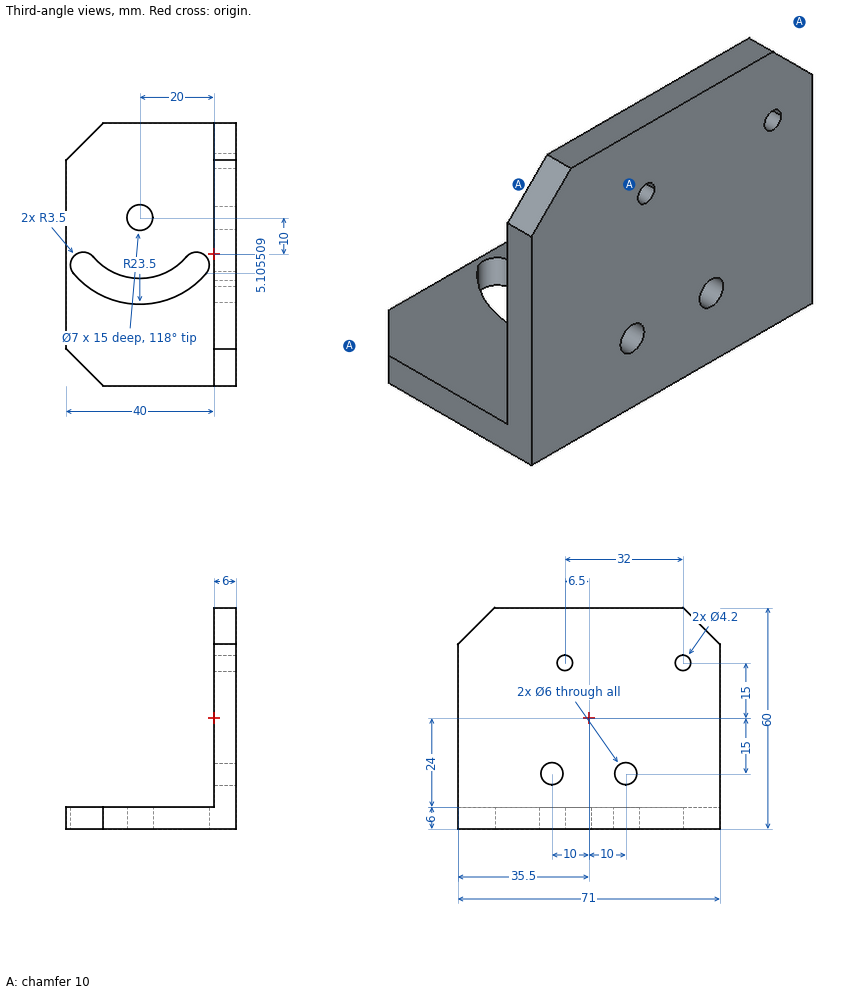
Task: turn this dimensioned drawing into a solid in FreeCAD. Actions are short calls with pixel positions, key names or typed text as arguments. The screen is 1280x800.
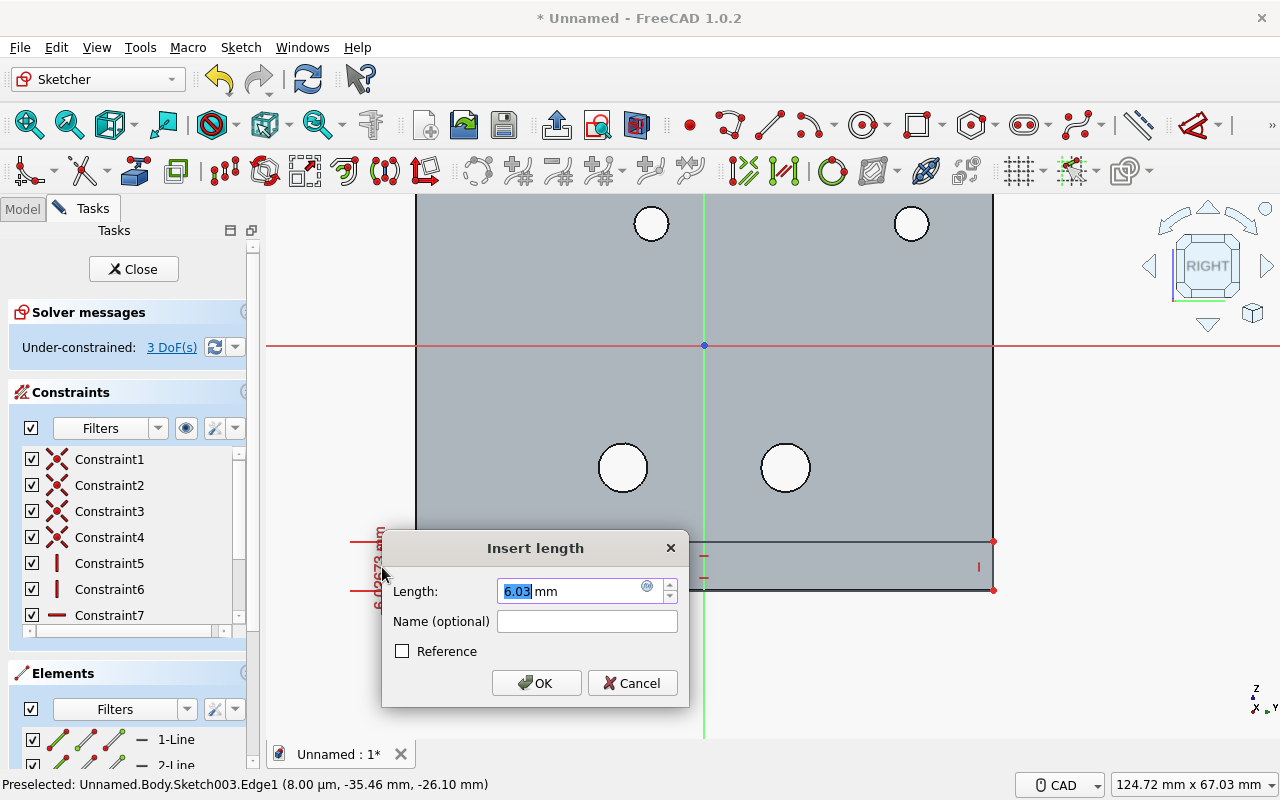
text(6)
key(Return)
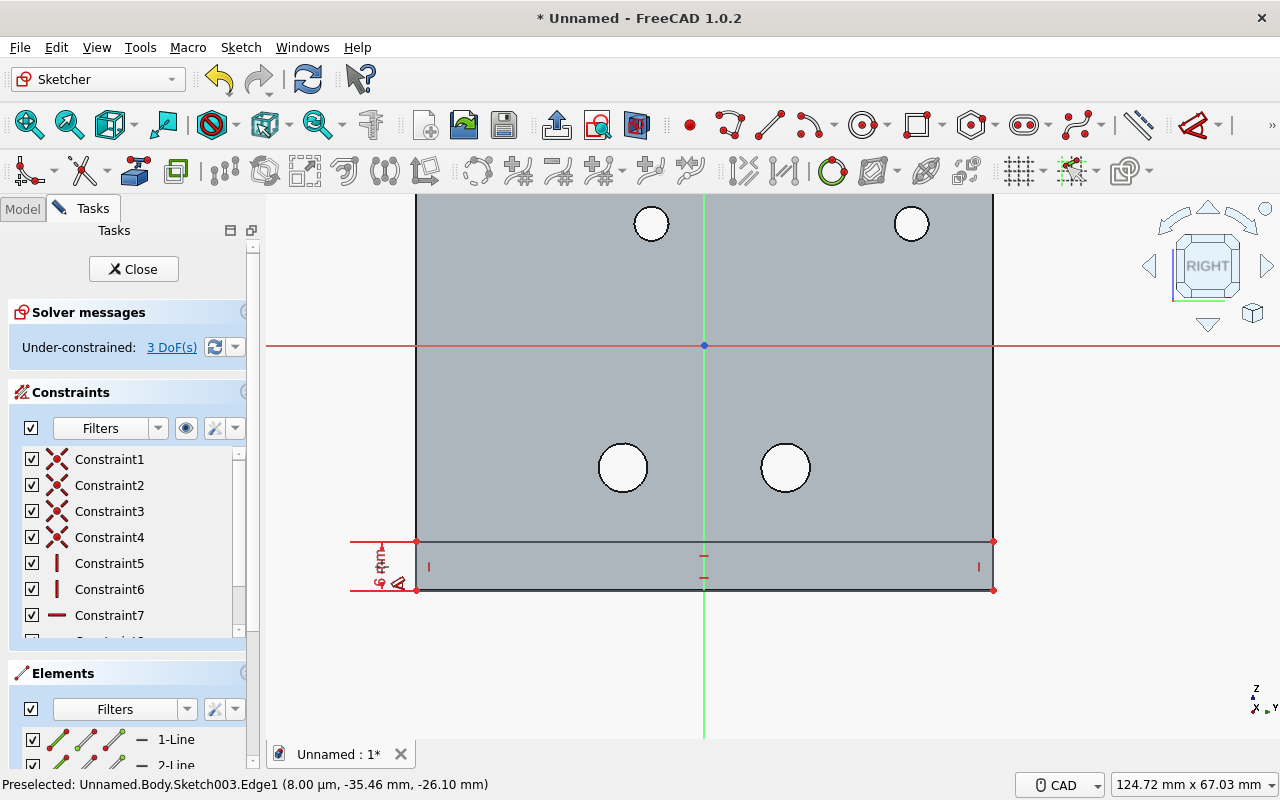
click(589, 591)
click(572, 625)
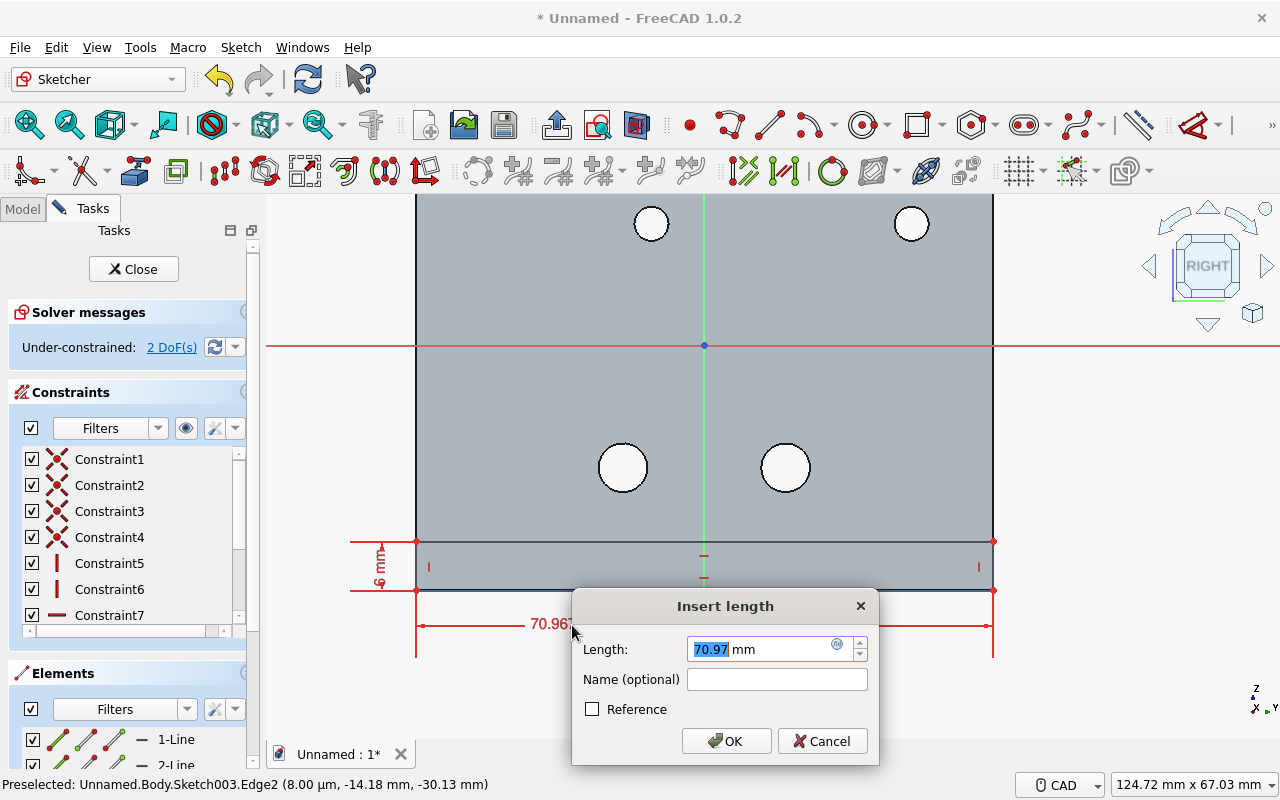
text(71)
key(Return)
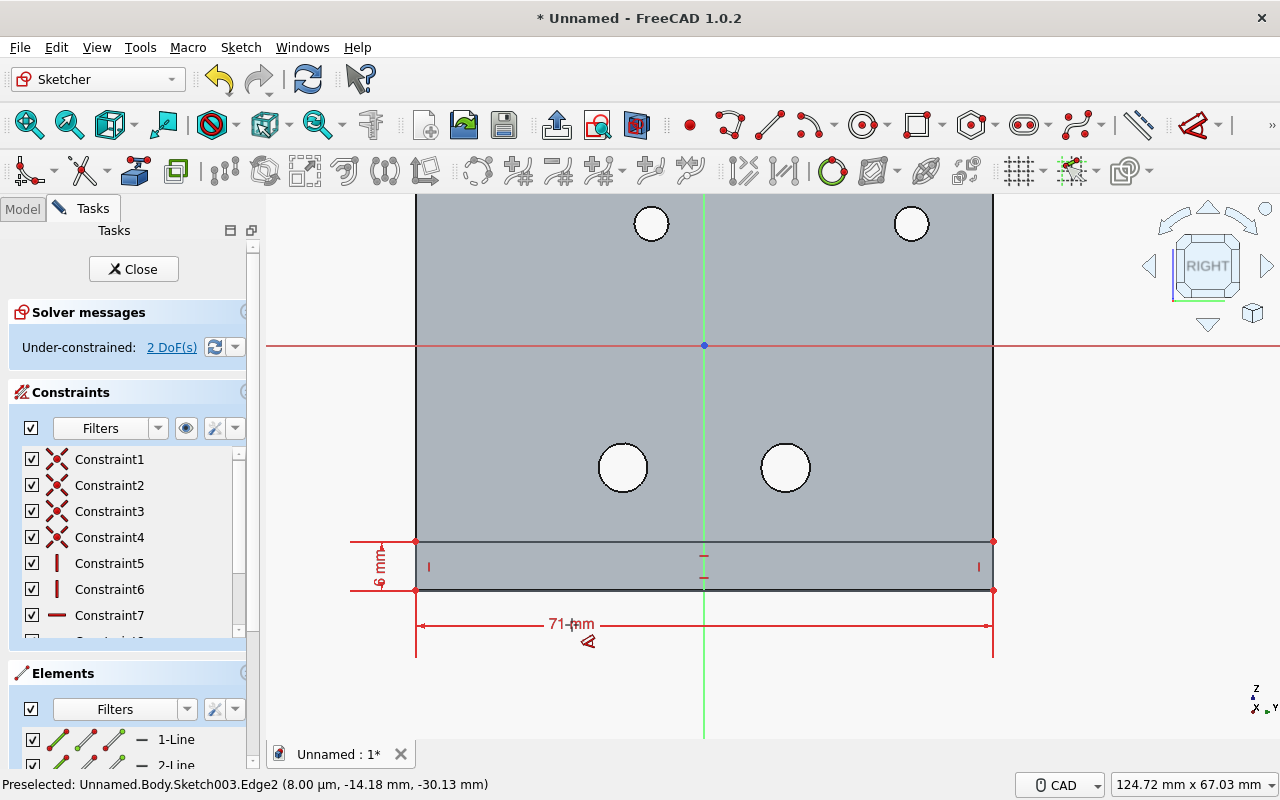
click(416, 542)
click(382, 444)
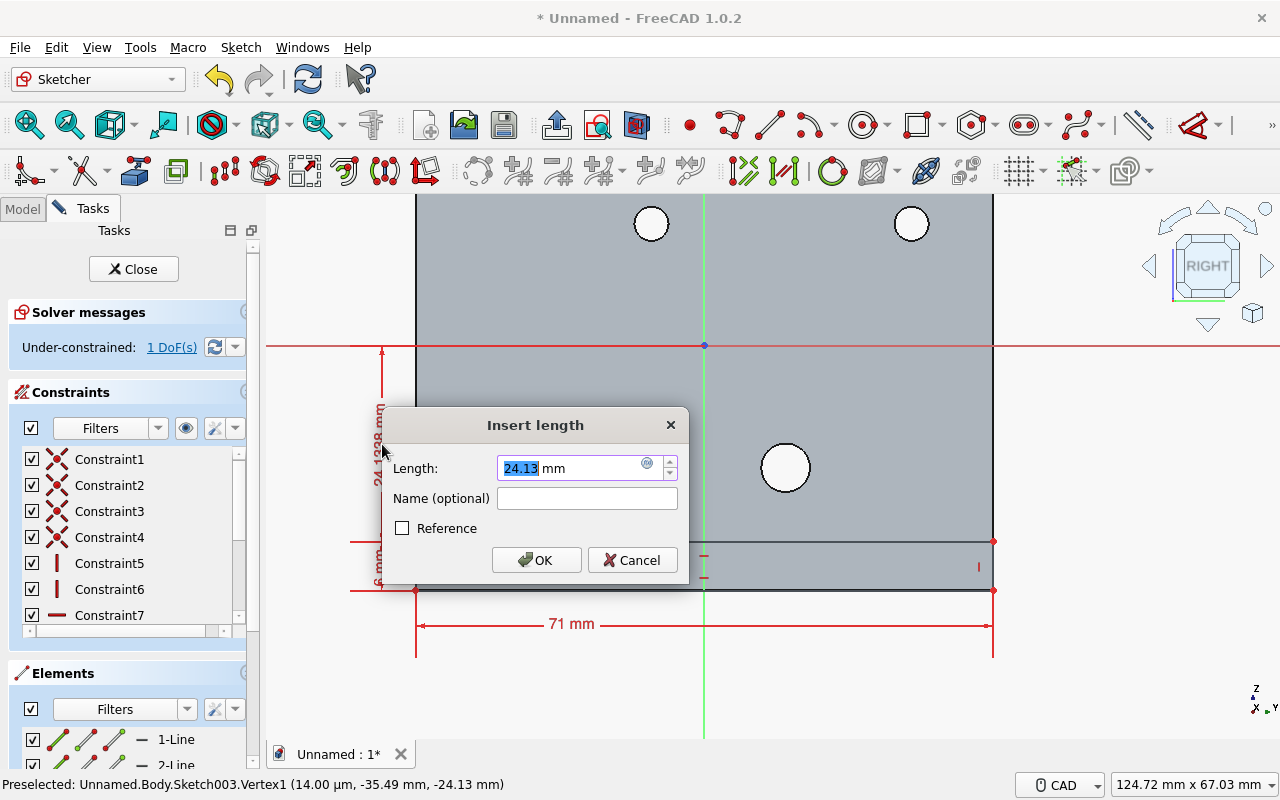
text(24)
key(Return)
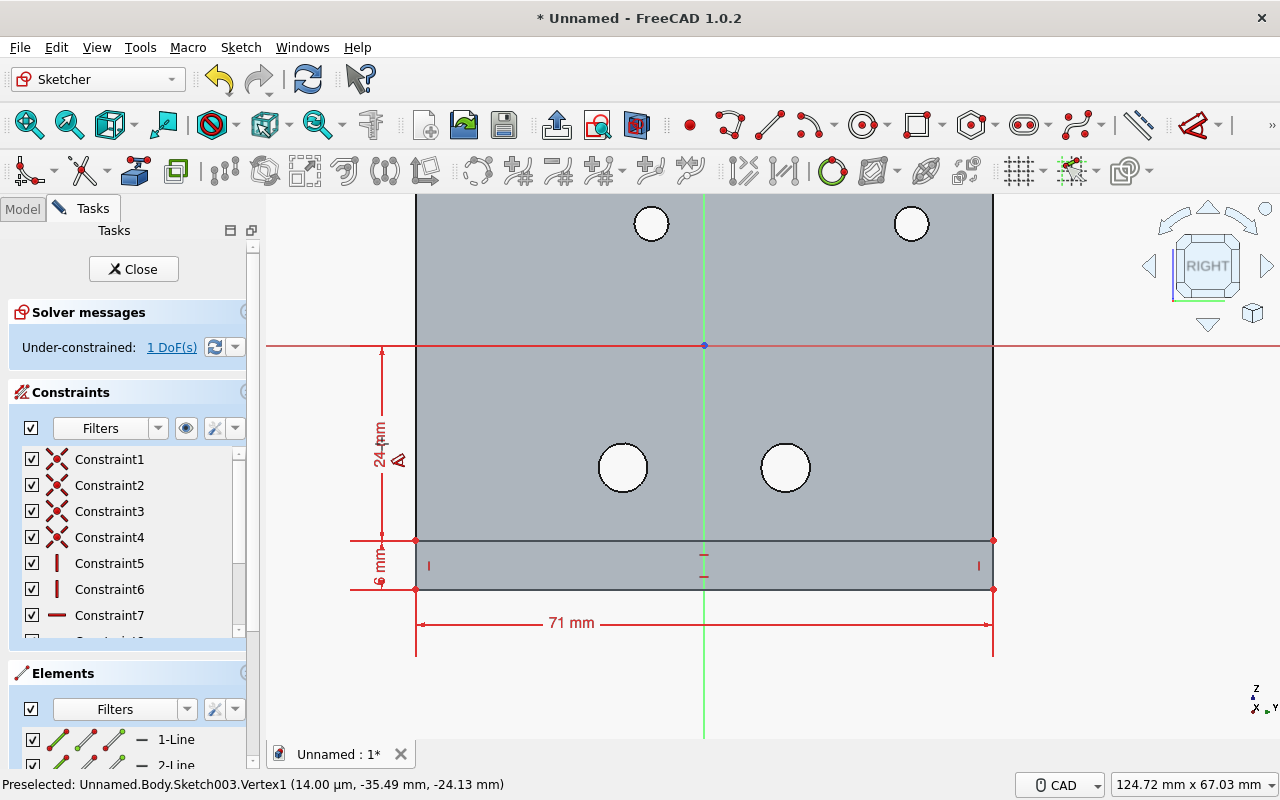
click(416, 541)
click(560, 312)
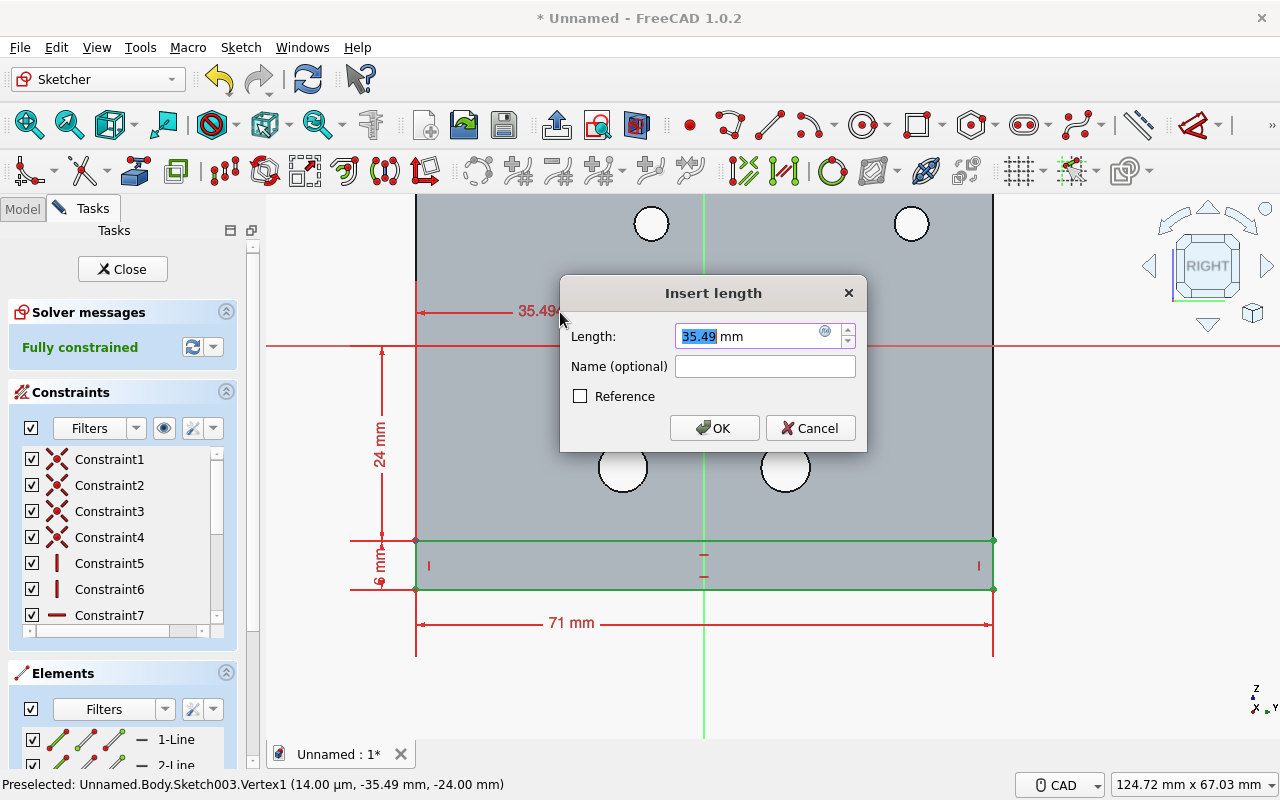
text(35.5)
key(Return)
key(Escape)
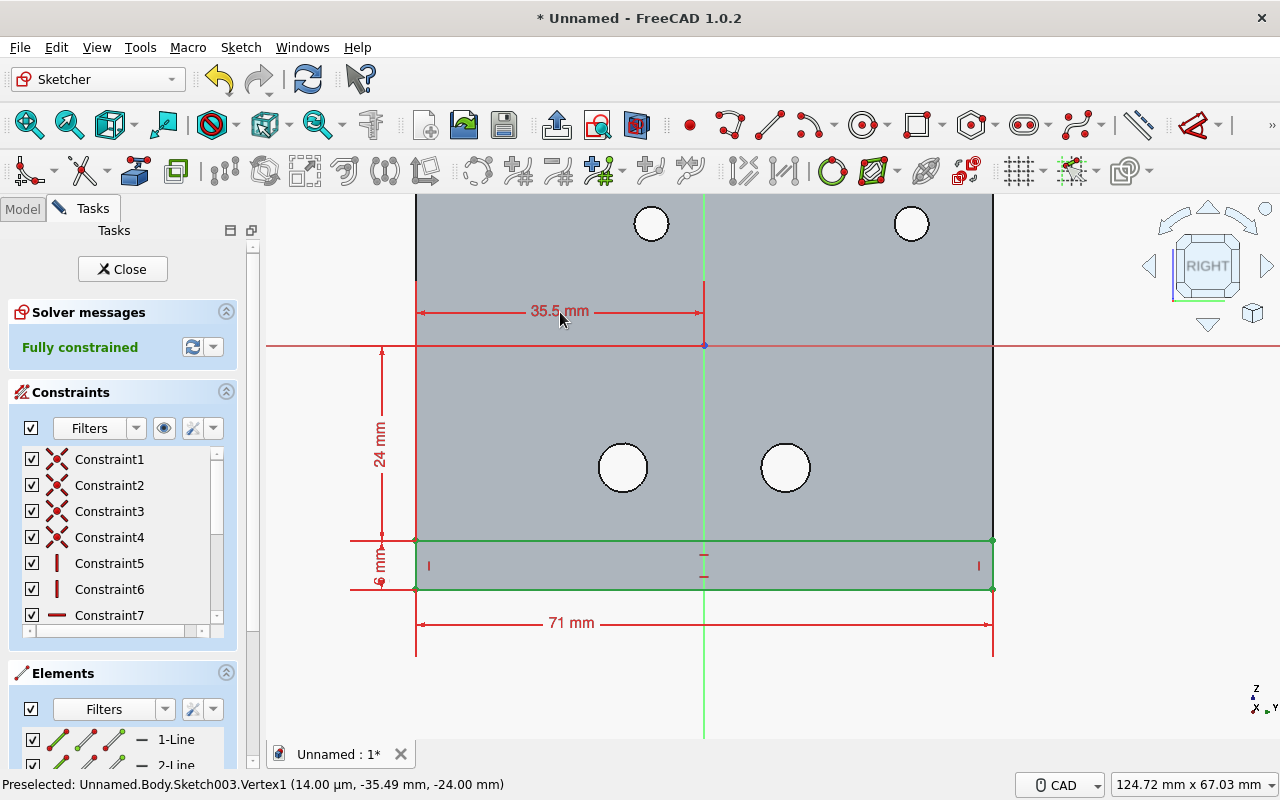
click(123, 269)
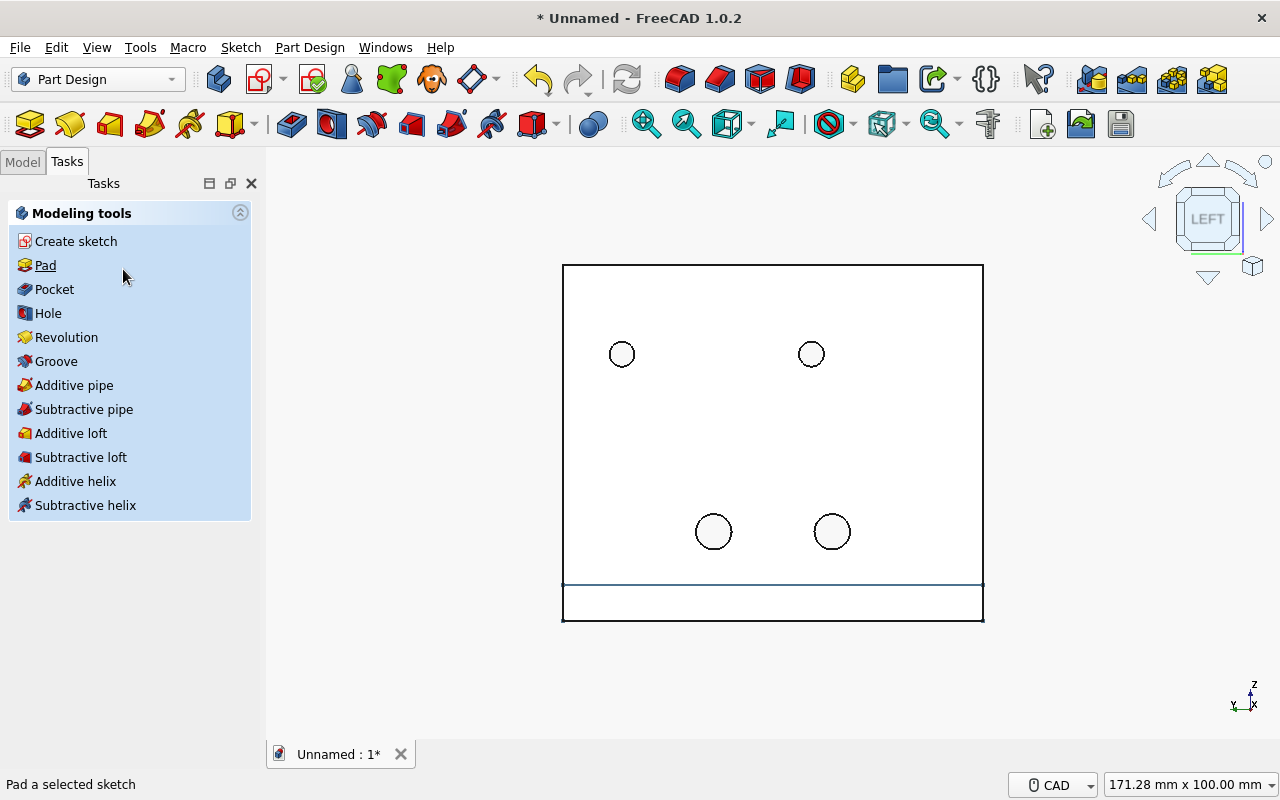
click(30, 124)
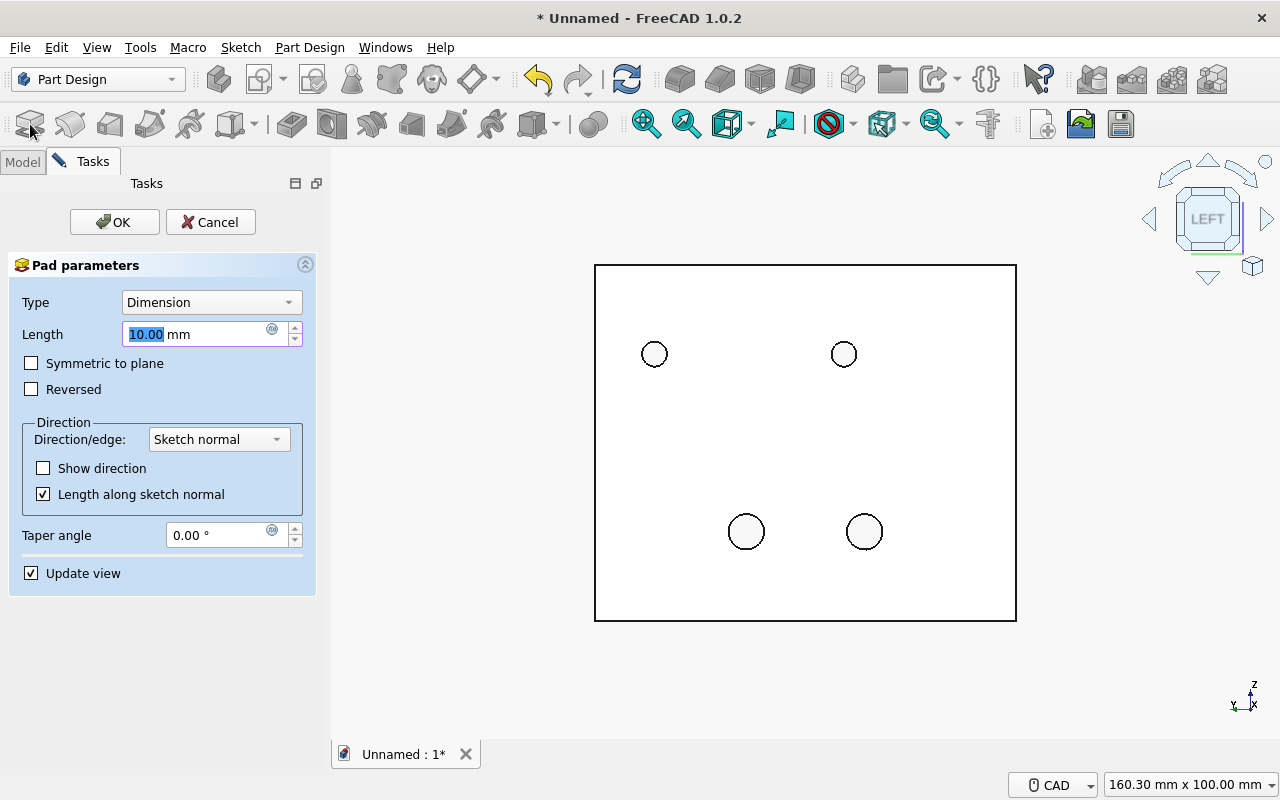
text(40)
key(Tab)